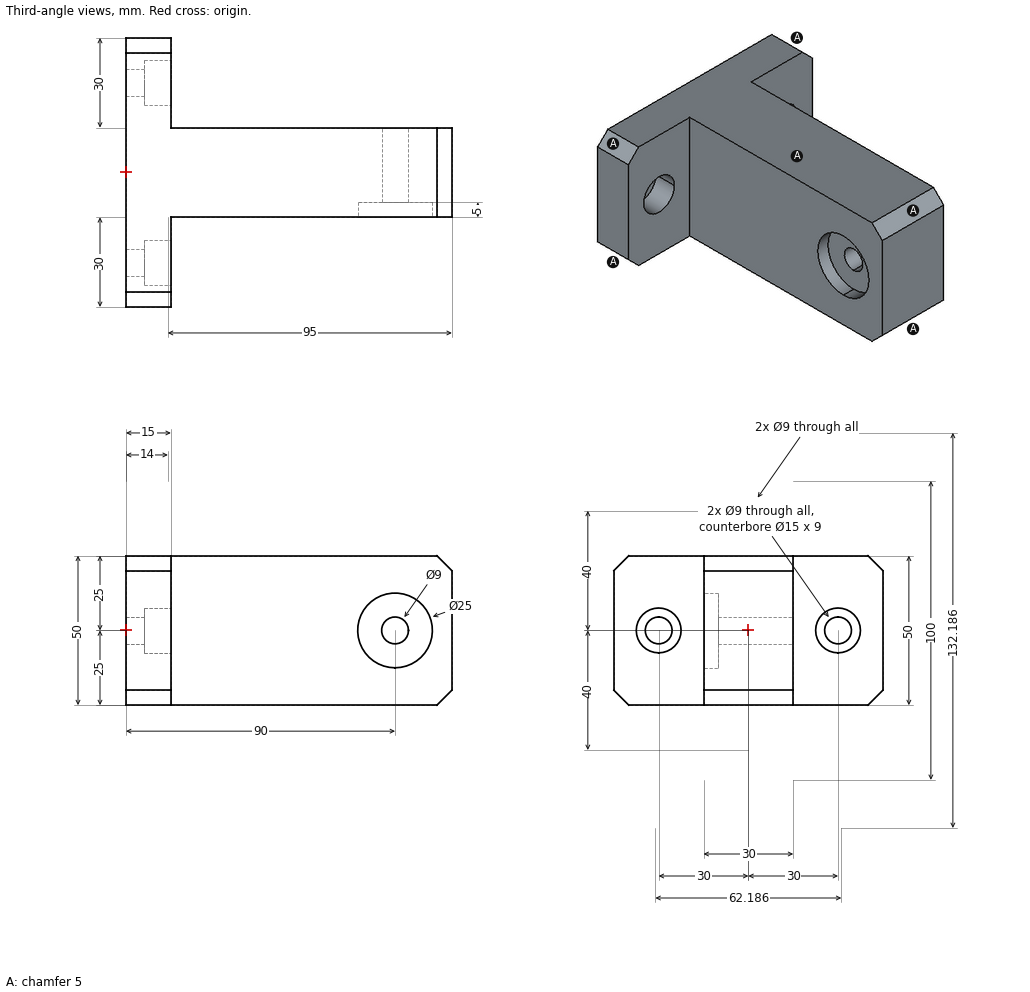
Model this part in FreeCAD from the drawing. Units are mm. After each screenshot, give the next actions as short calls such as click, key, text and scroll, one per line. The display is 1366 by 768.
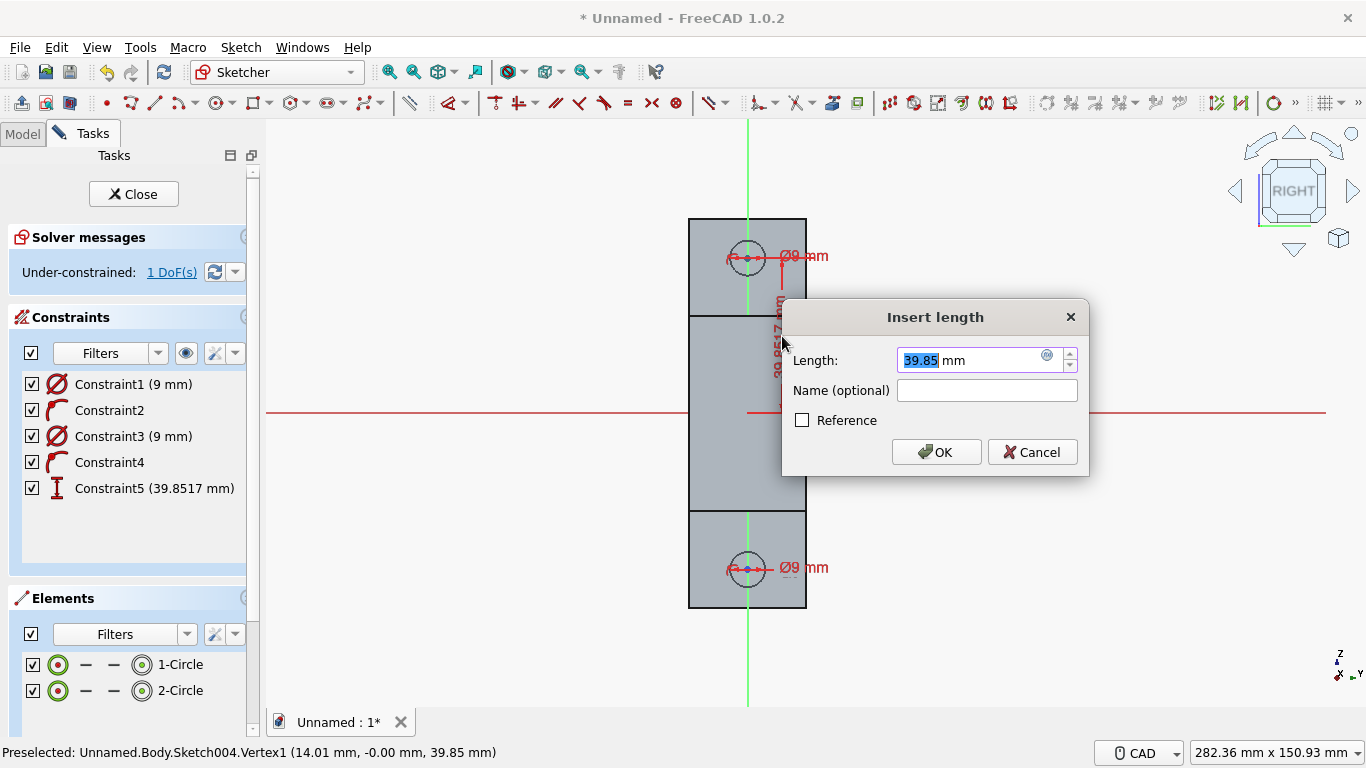
text(40)
key(Return)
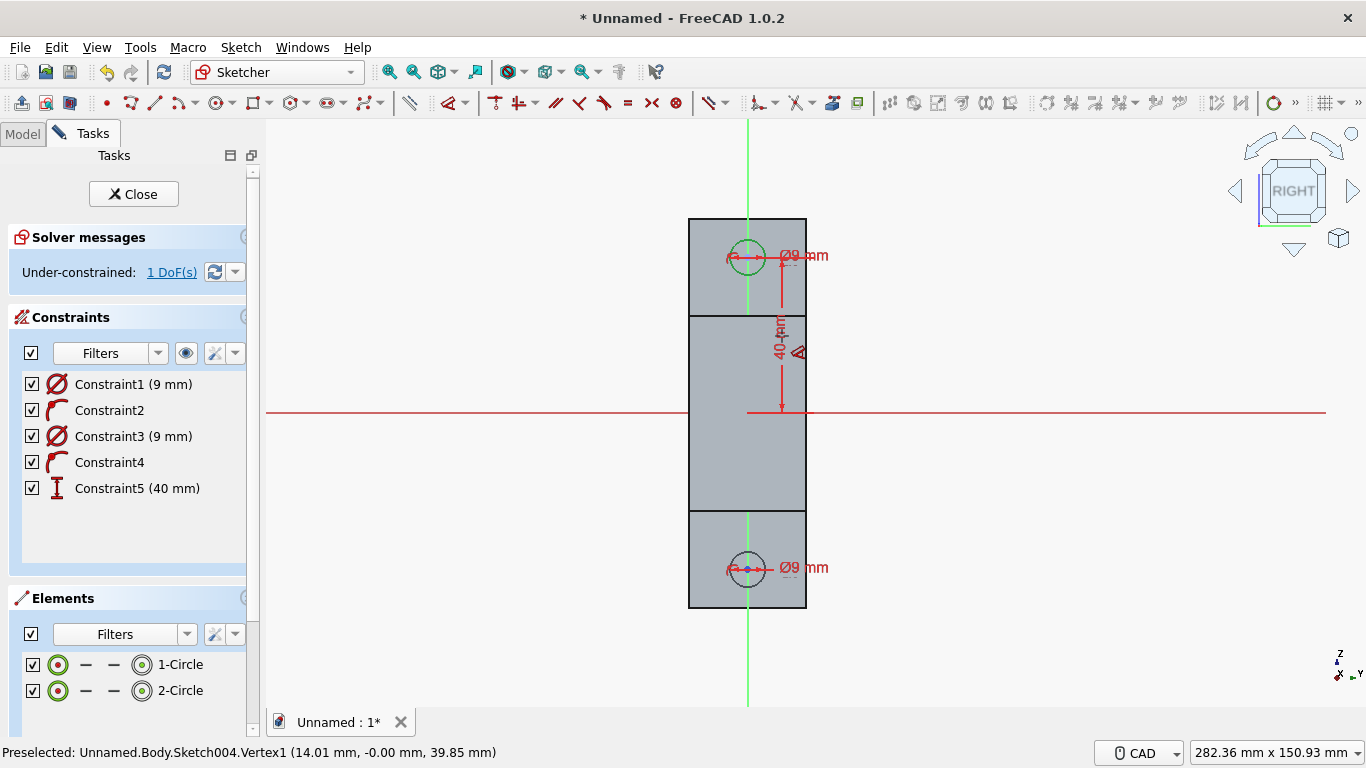
click(748, 570)
click(782, 491)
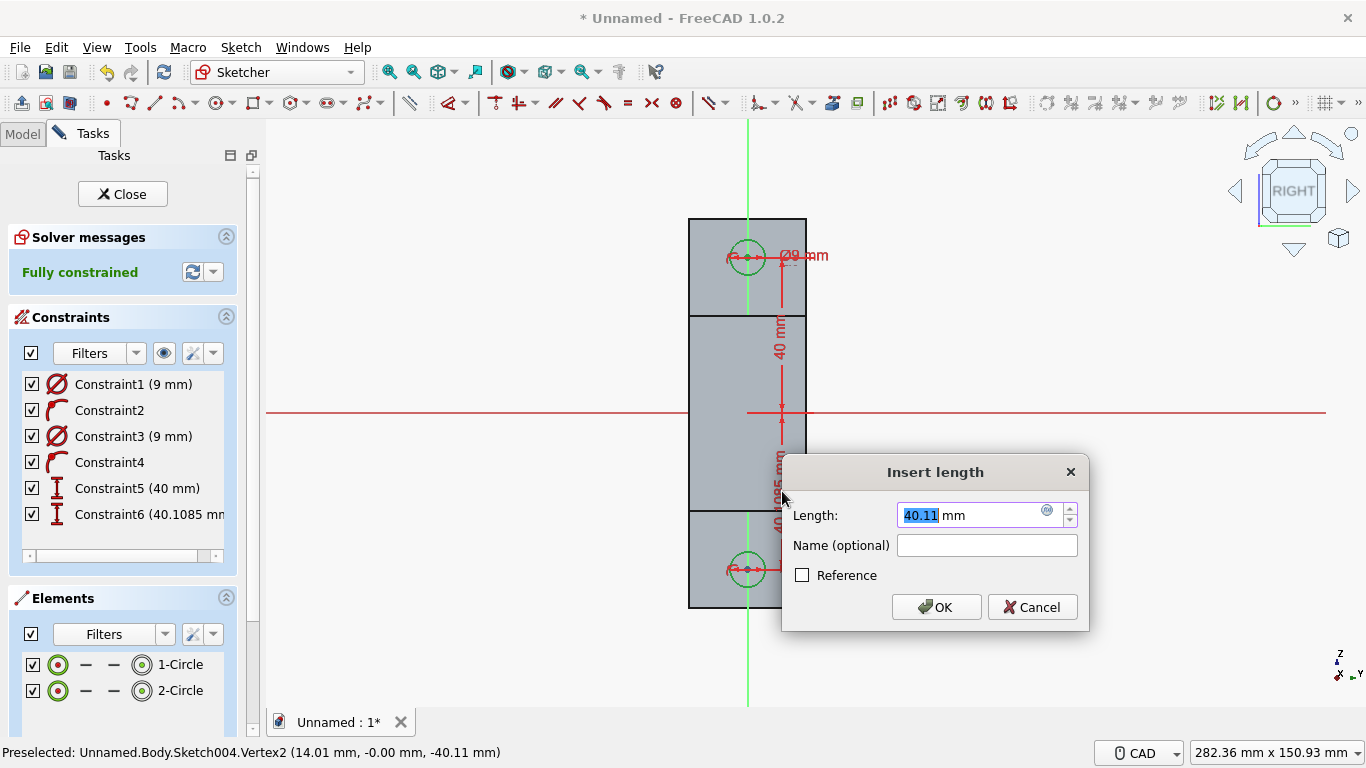
text(40)
key(Return)
key(Escape)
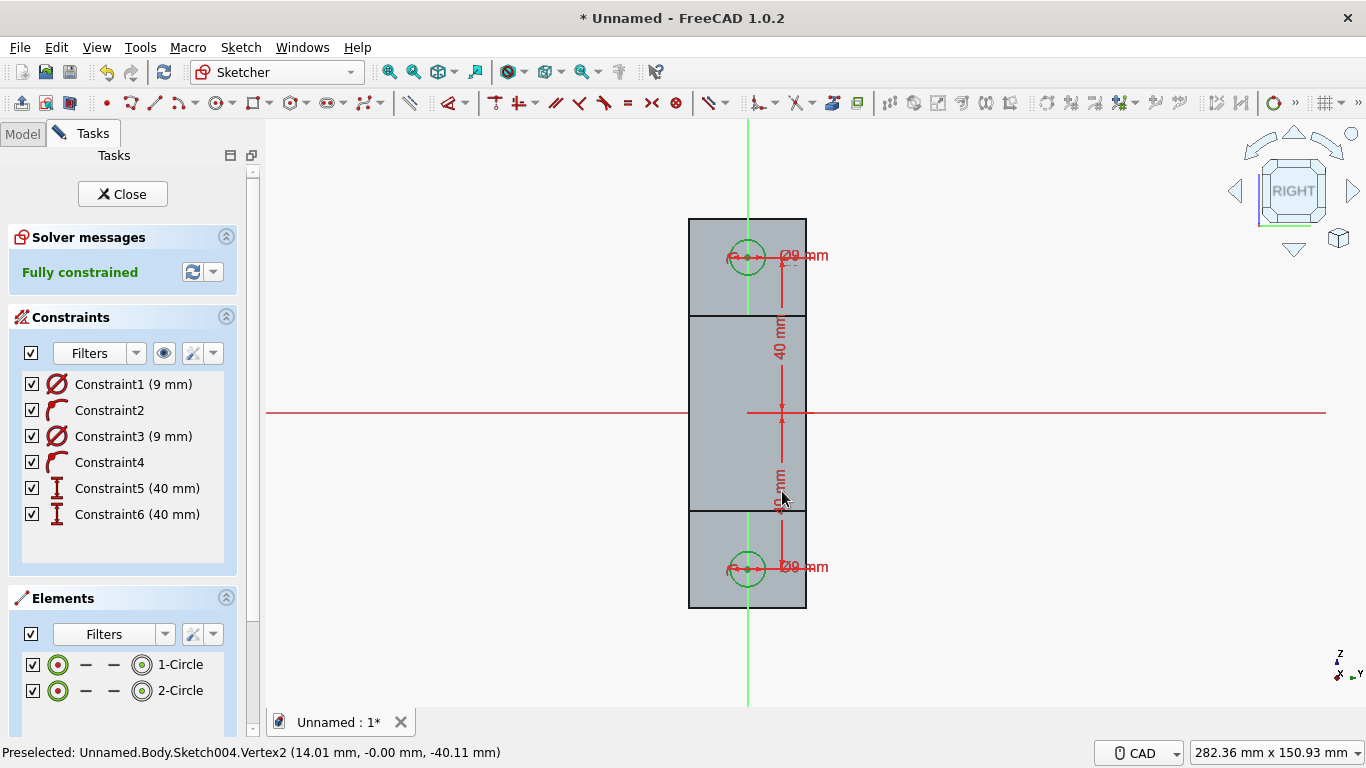
click(123, 194)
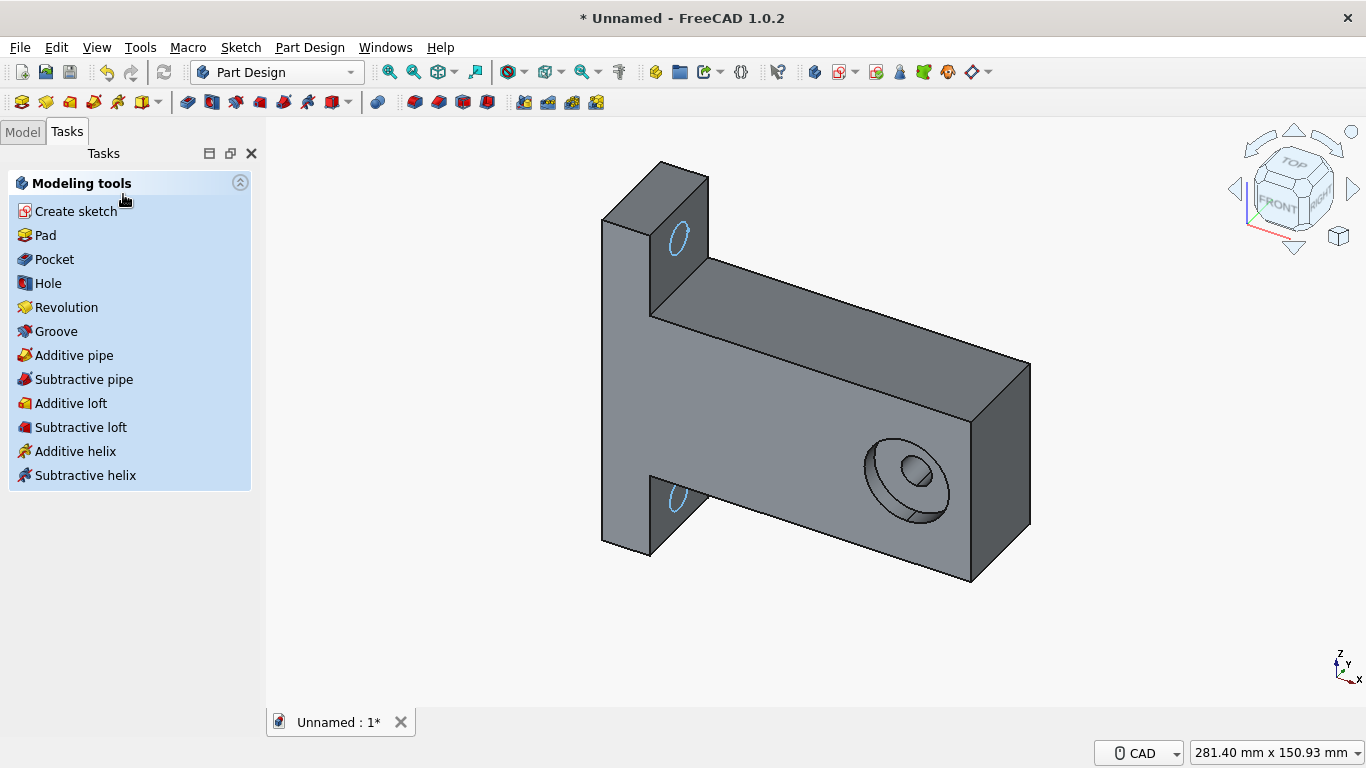
click(212, 102)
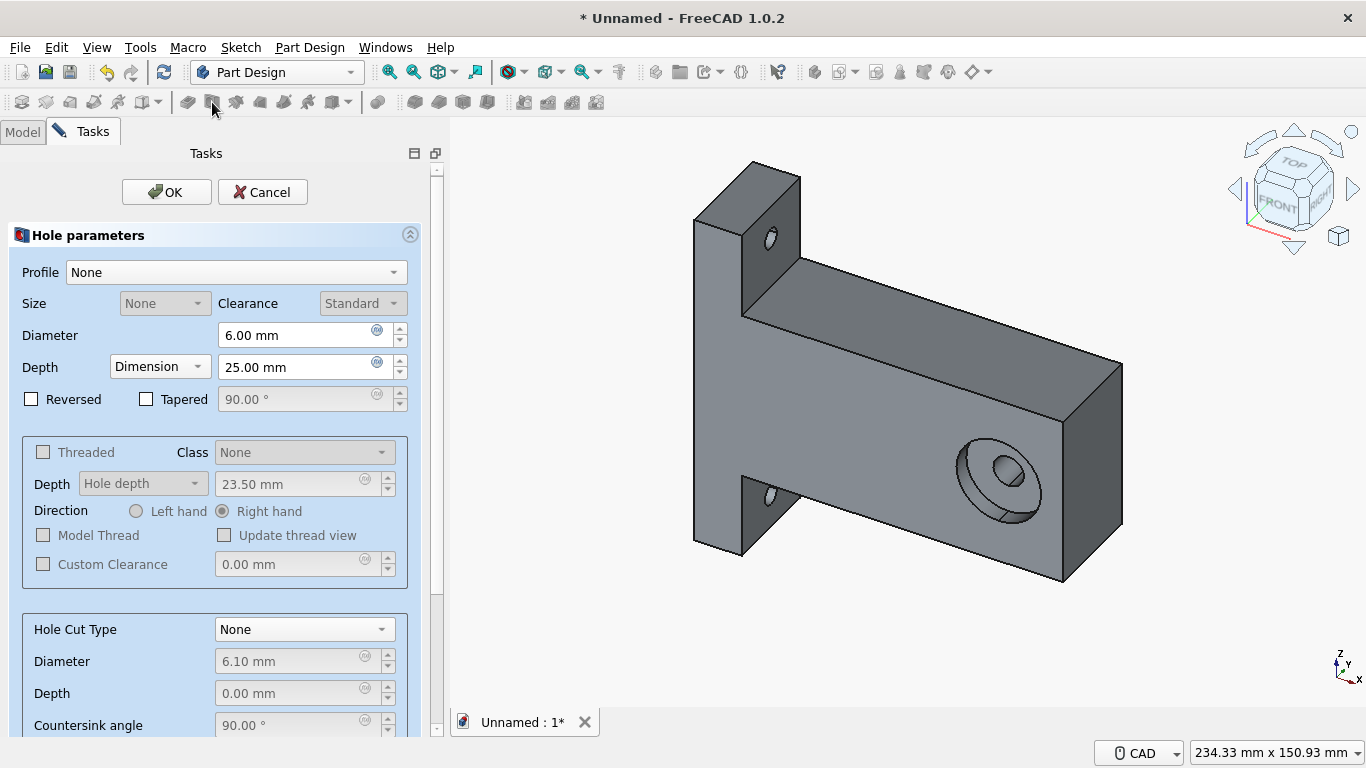
triple_click(305, 335)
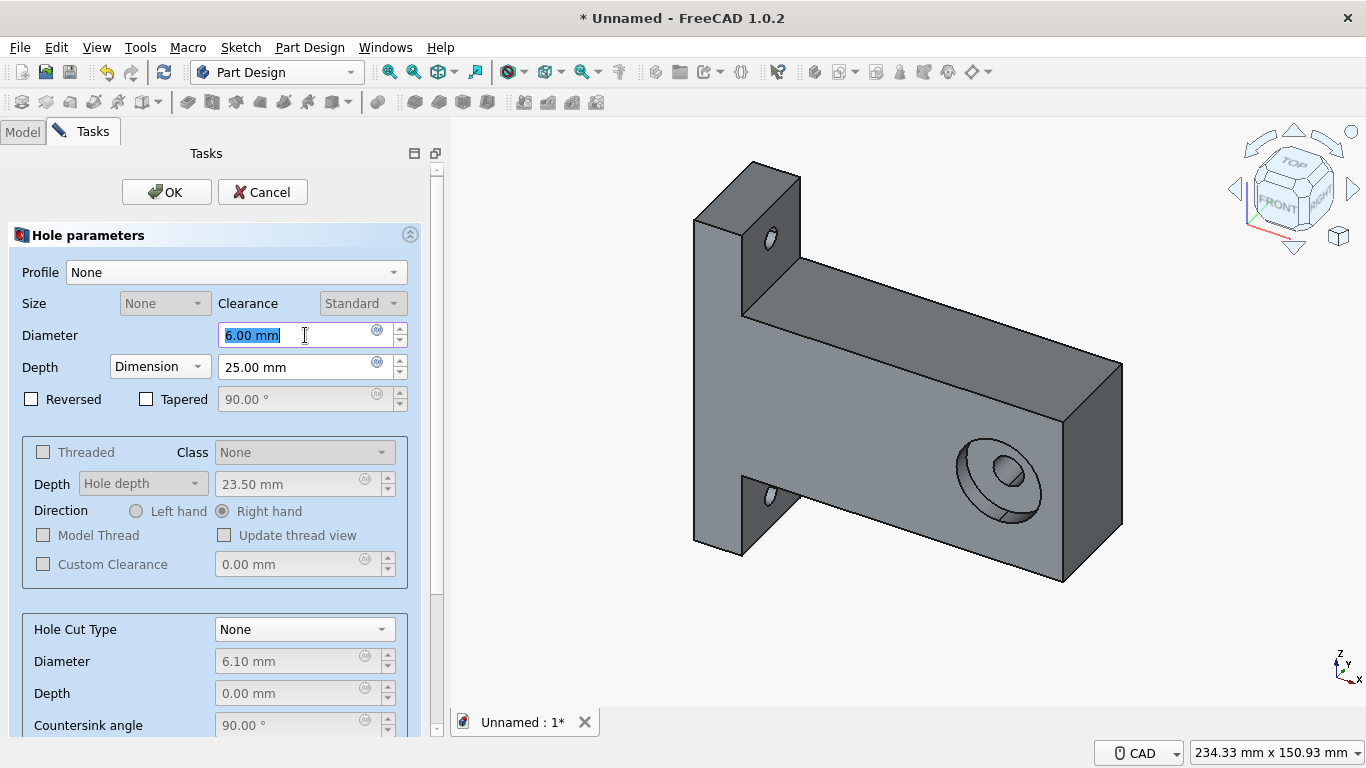
text(9)
key(Tab)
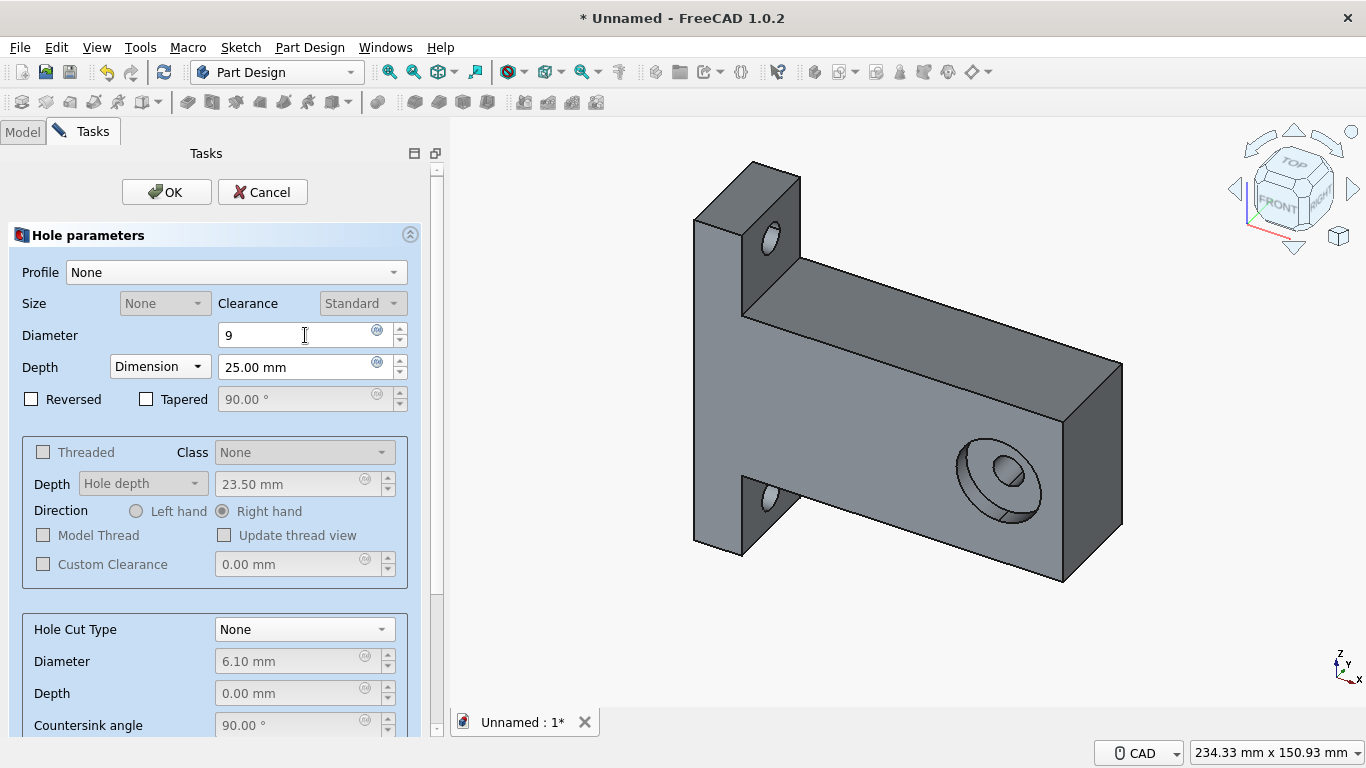
click(161, 366)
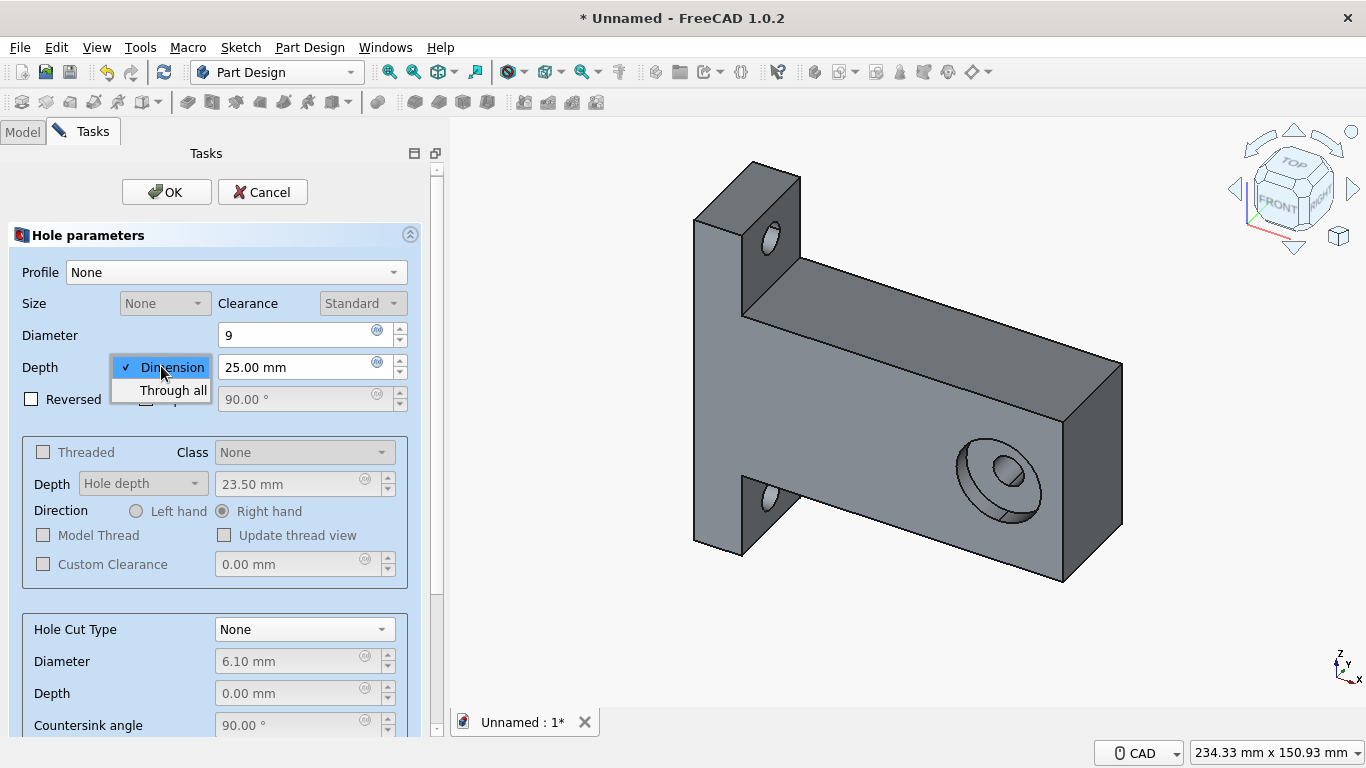
click(160, 390)